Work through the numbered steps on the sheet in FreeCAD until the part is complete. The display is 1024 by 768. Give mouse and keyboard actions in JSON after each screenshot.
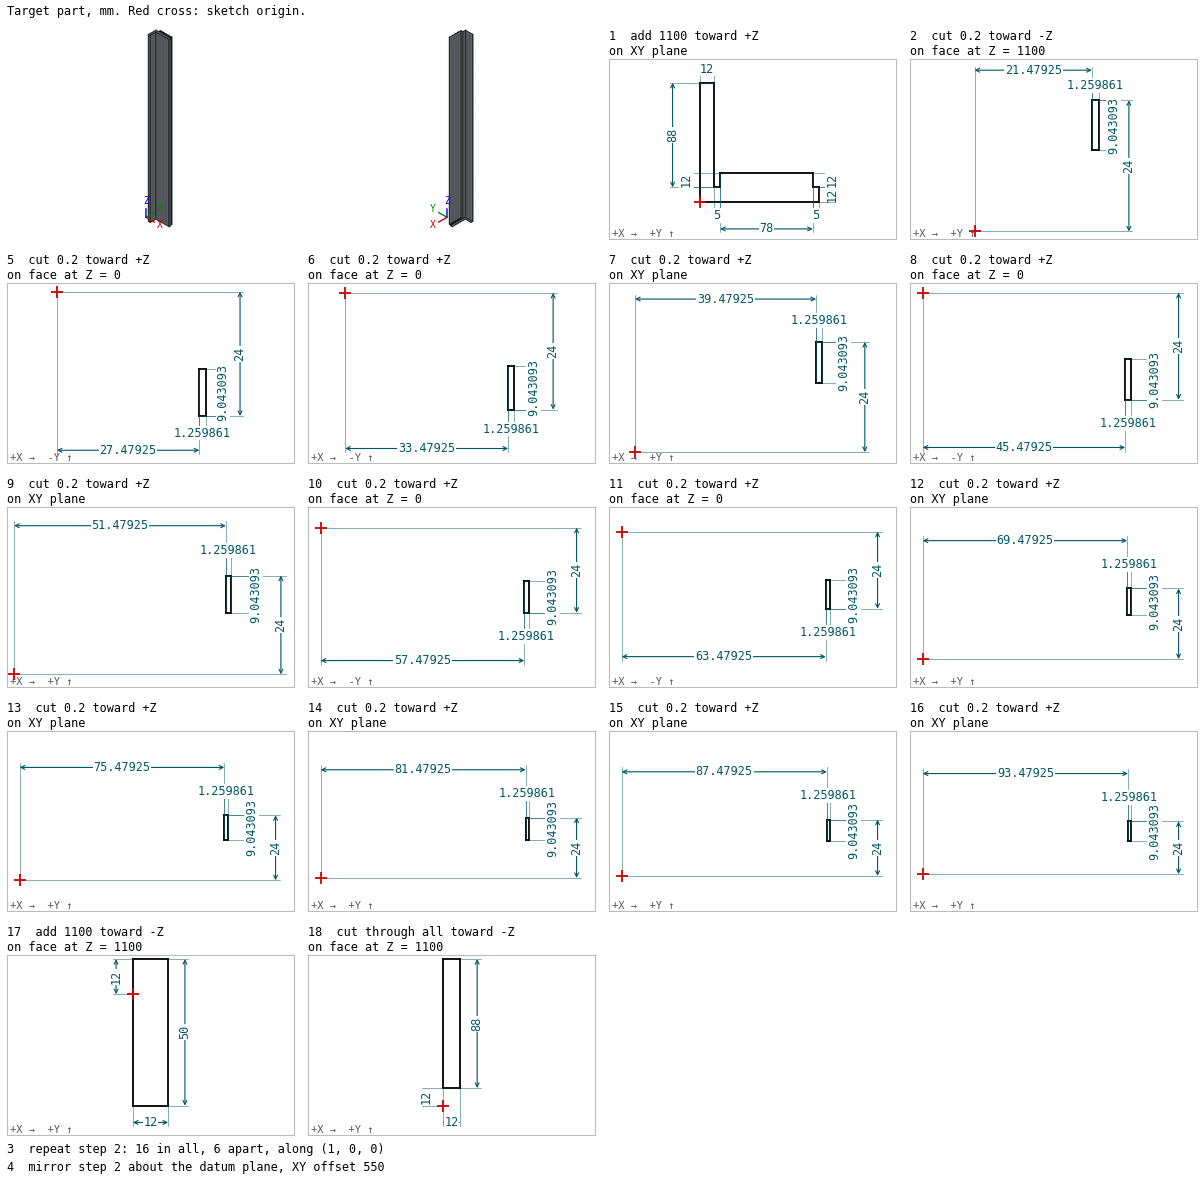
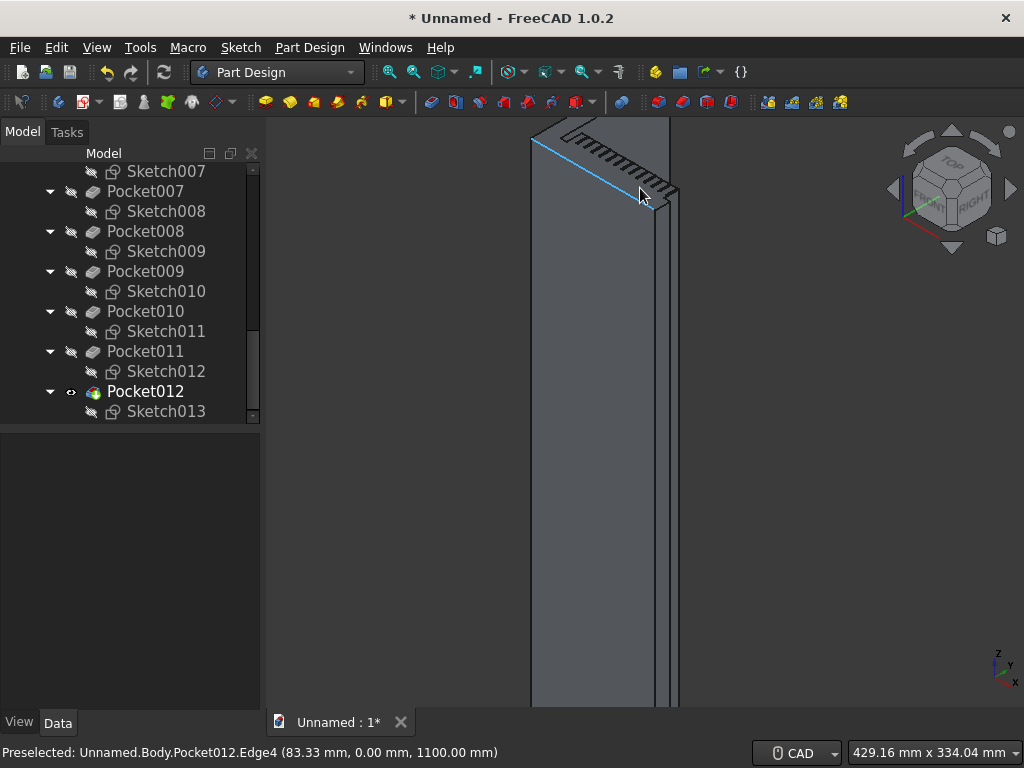
{"action": "left_click", "coordinate": [620, 178]}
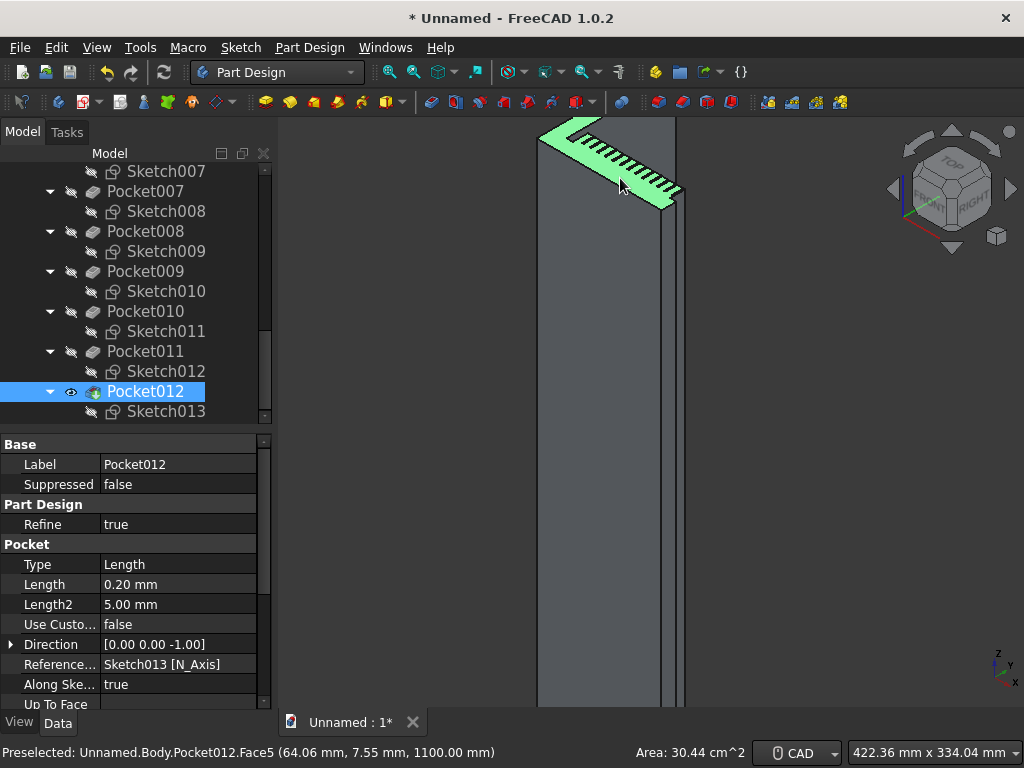
{"action": "left_click", "coordinate": [84, 102]}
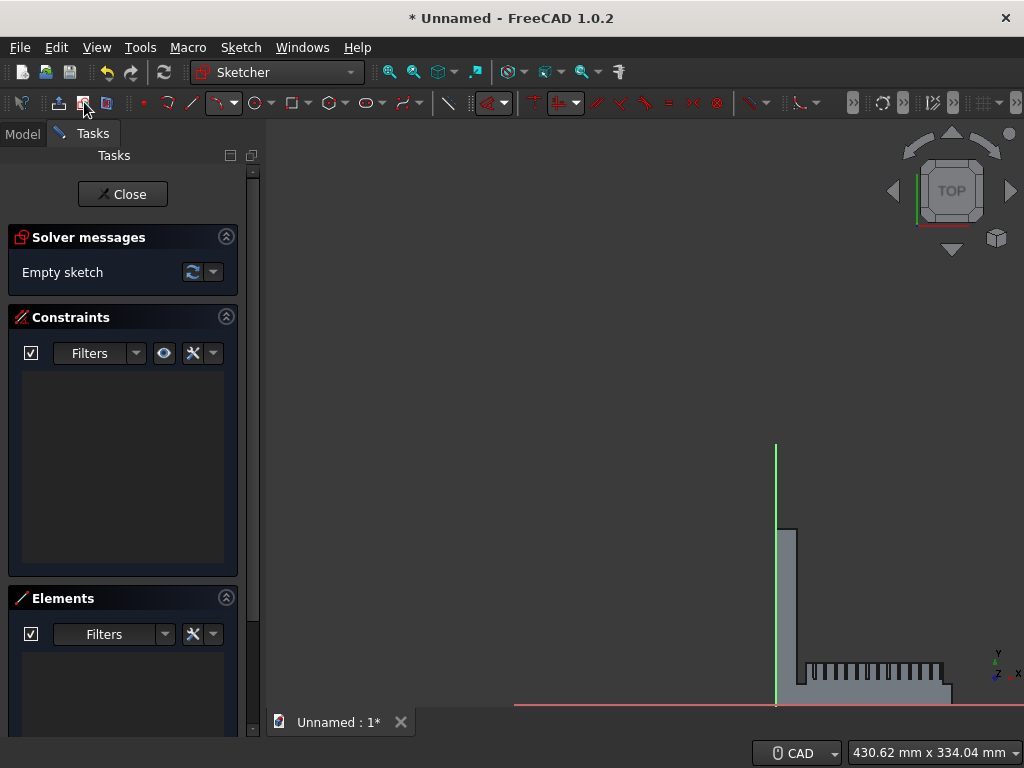
{"action": "scroll", "coordinate": [576, 413], "scroll_direction": "down", "scroll_amount": 5}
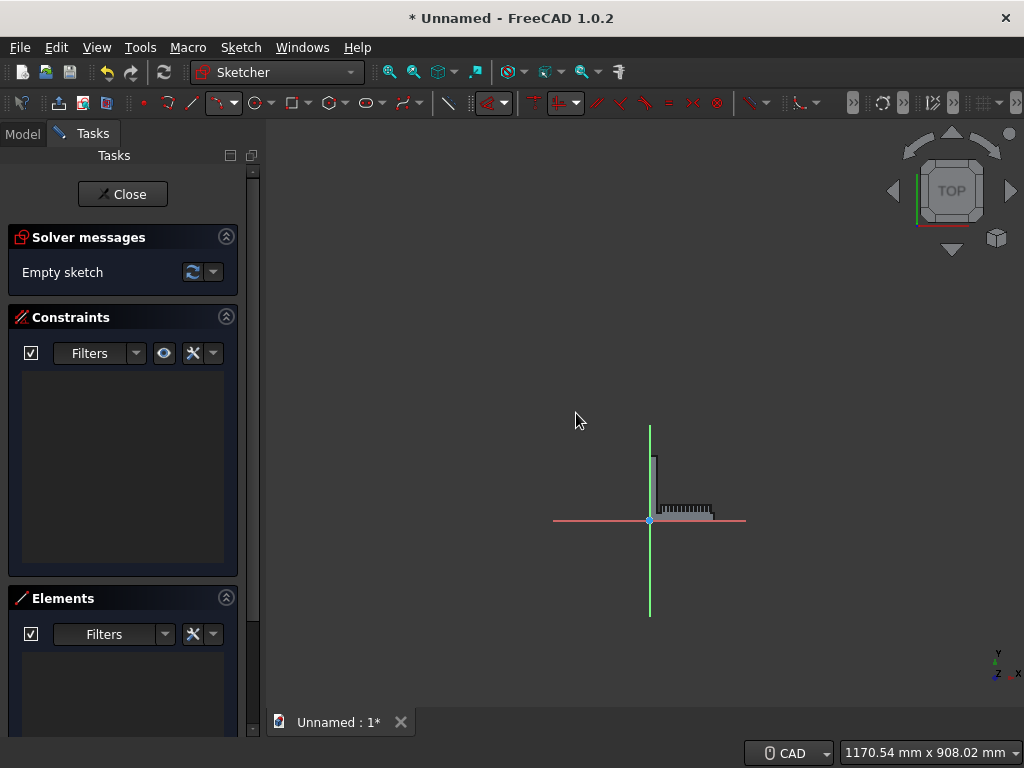
{"action": "scroll", "coordinate": [661, 541], "scroll_direction": "up", "scroll_amount": 12}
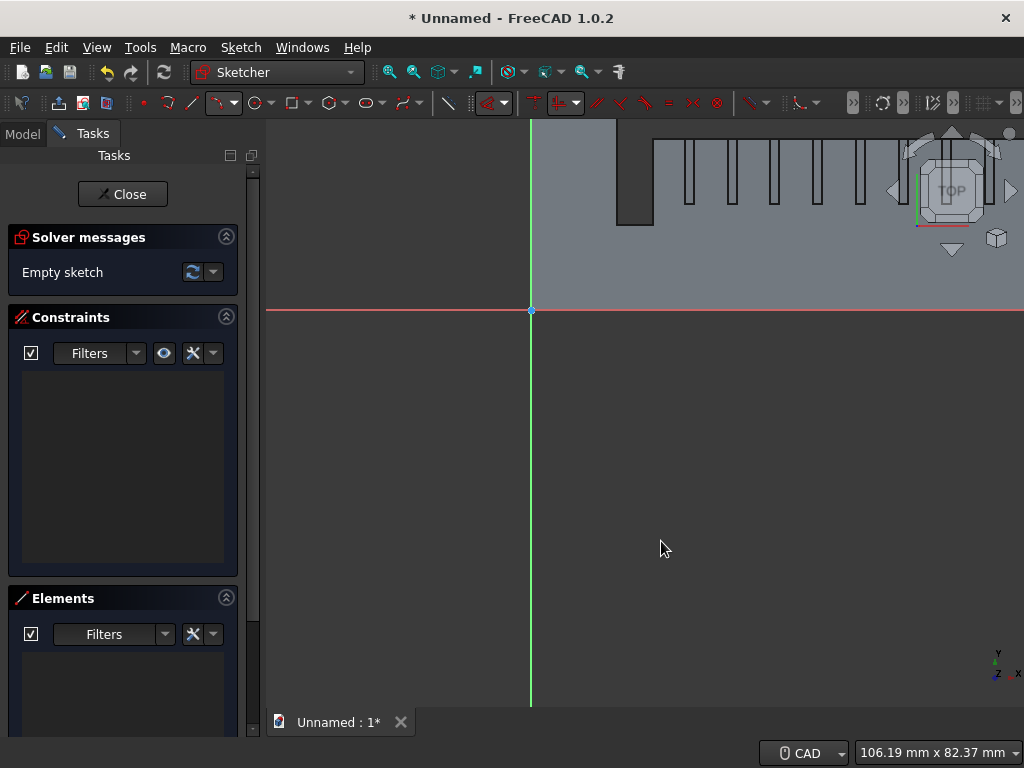
{"action": "key", "text": "g r"}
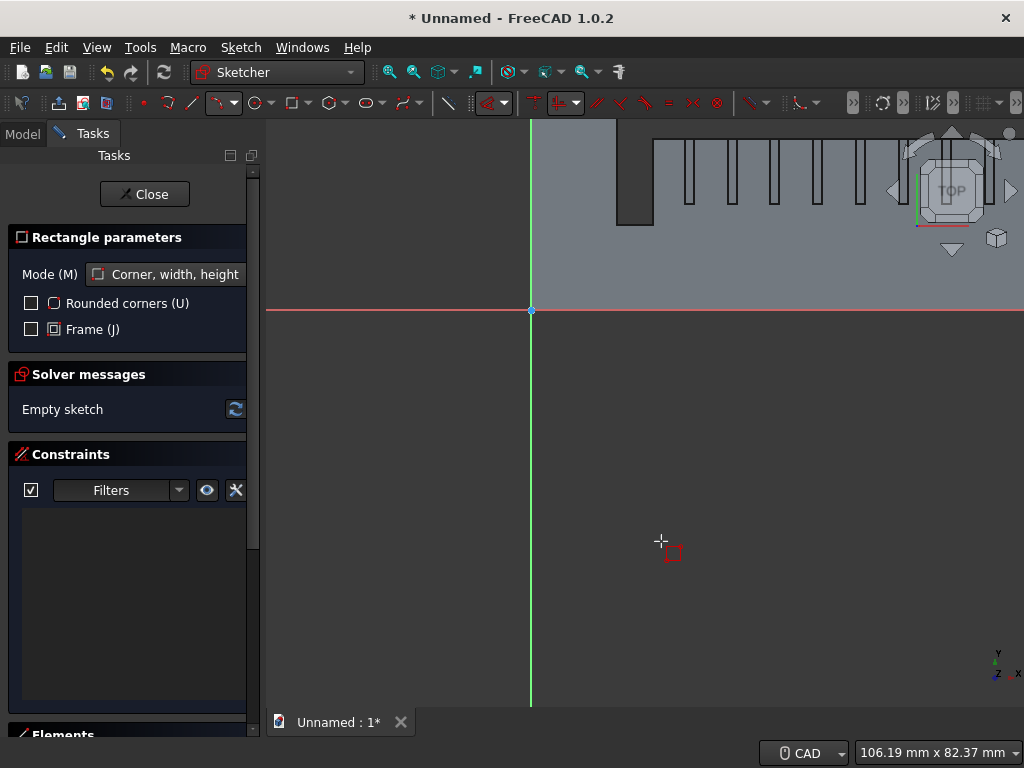
{"action": "left_click", "coordinate": [531, 225]}
{"action": "mouse_move", "coordinate": [617, 582]}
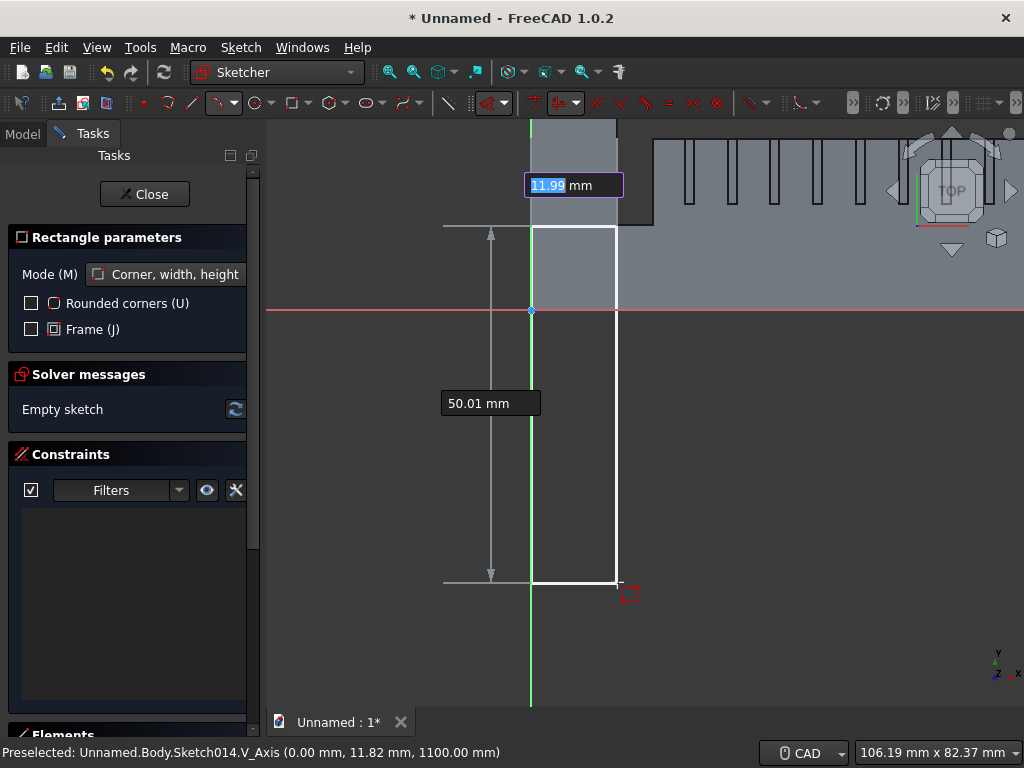
{"action": "type", "text": "12"}
{"action": "key", "text": "Tab"}
{"action": "type", "text": "50"}
{"action": "key", "text": "Return"}
{"action": "key", "text": "Escape"}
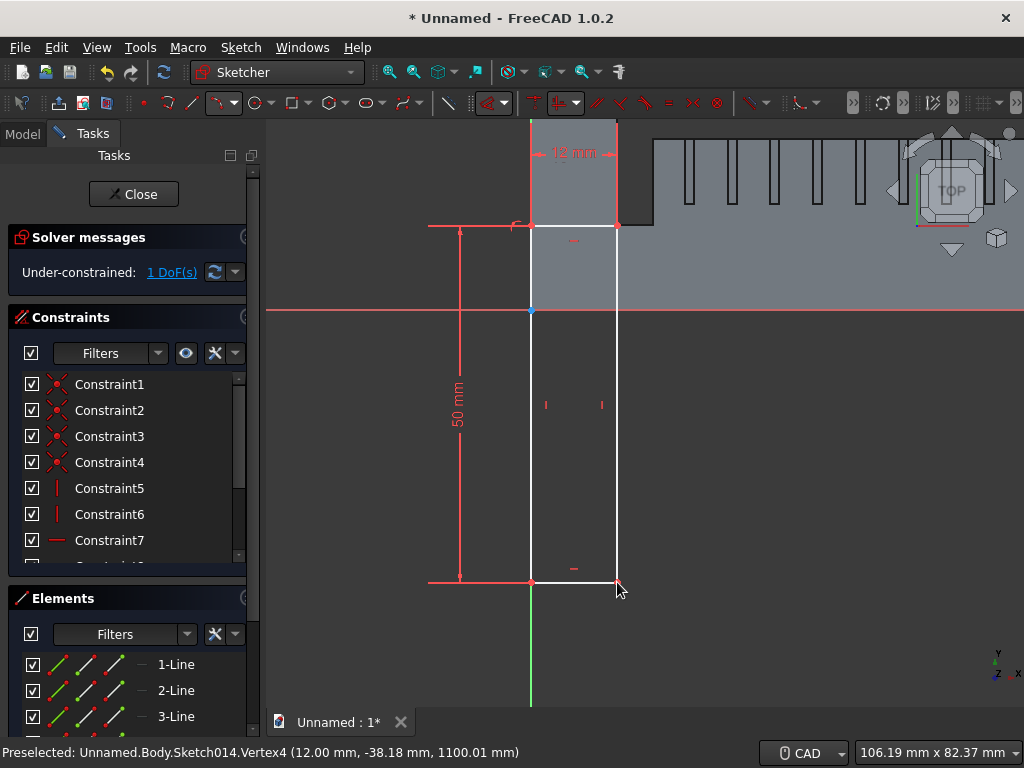
{"action": "left_click", "coordinate": [531, 226]}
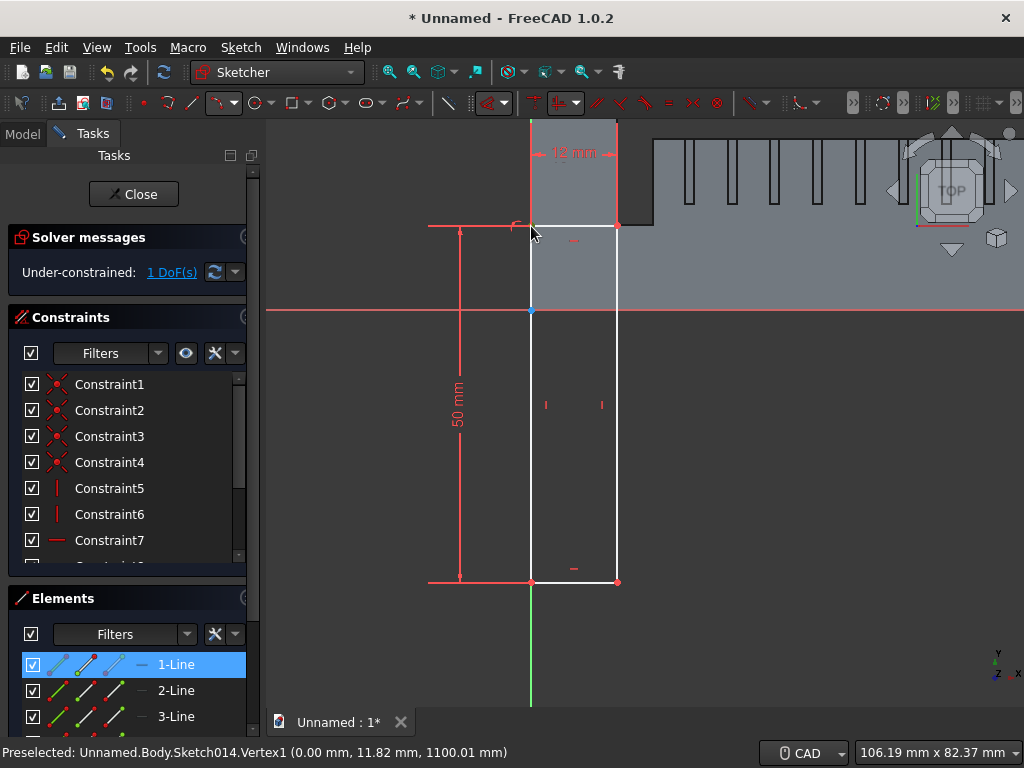
{"action": "left_click", "coordinate": [506, 104]}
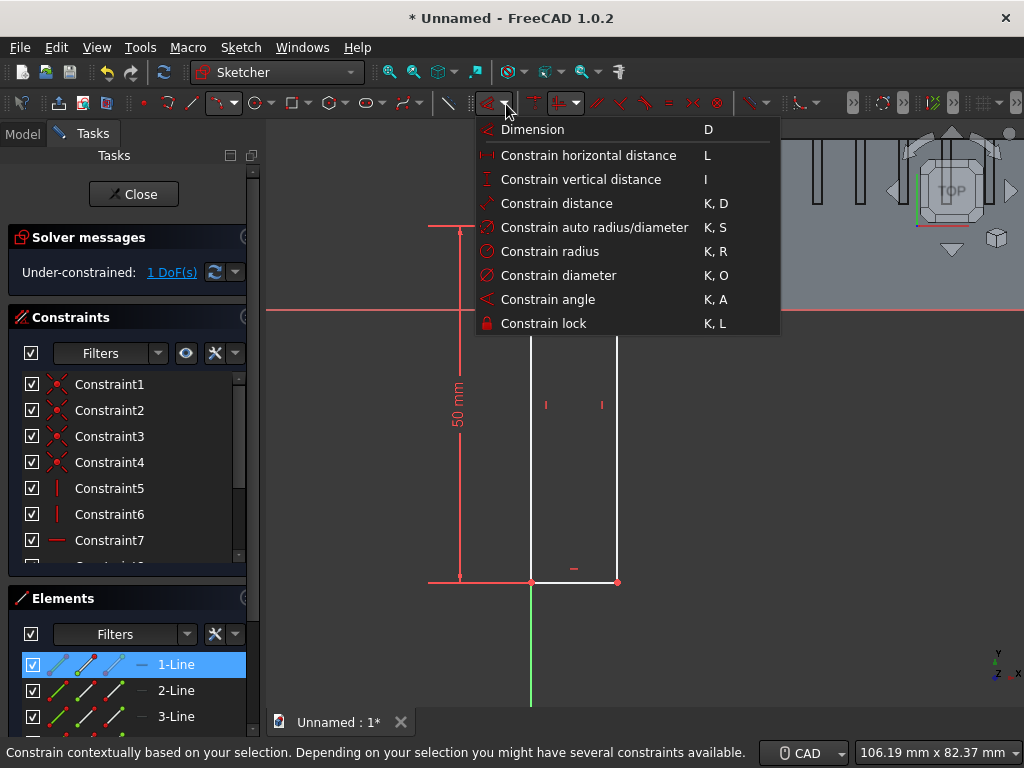
{"action": "left_click", "coordinate": [628, 179]}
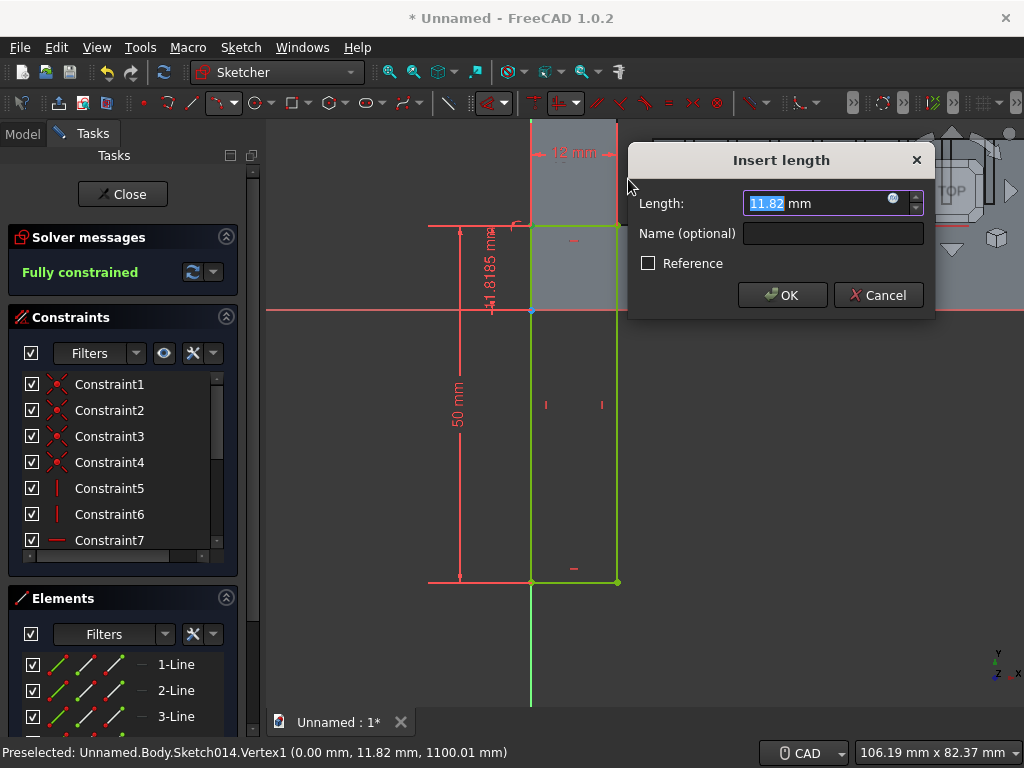
{"action": "type", "text": "12"}
{"action": "key", "text": "Return"}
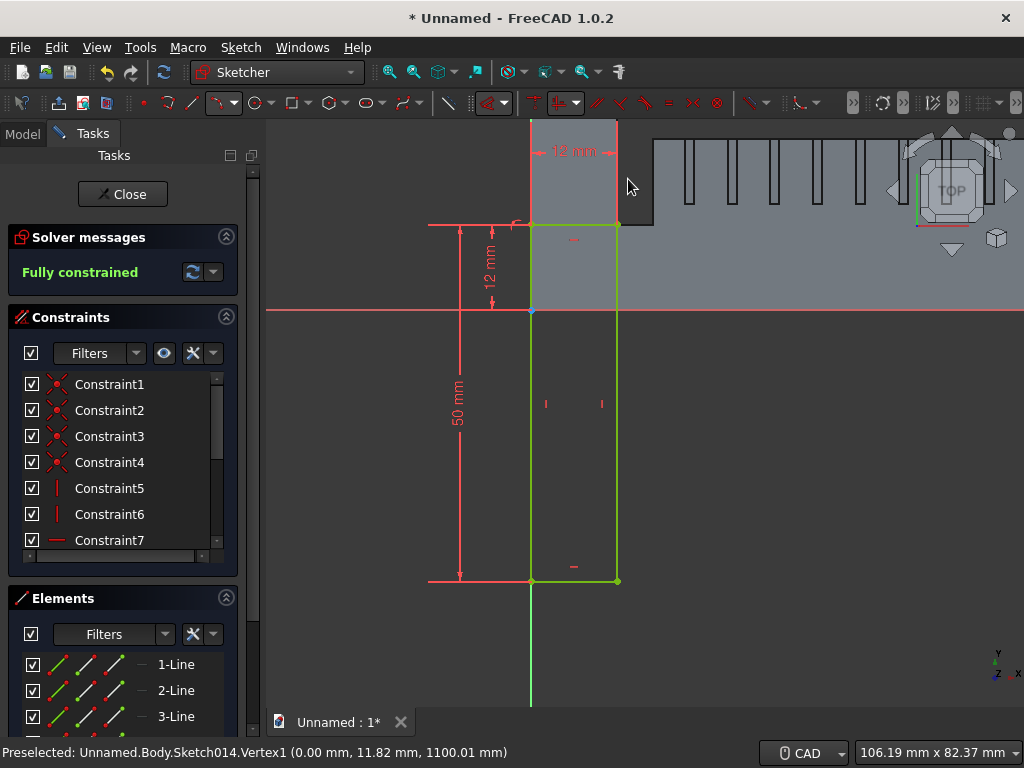
{"action": "left_click", "coordinate": [123, 194]}